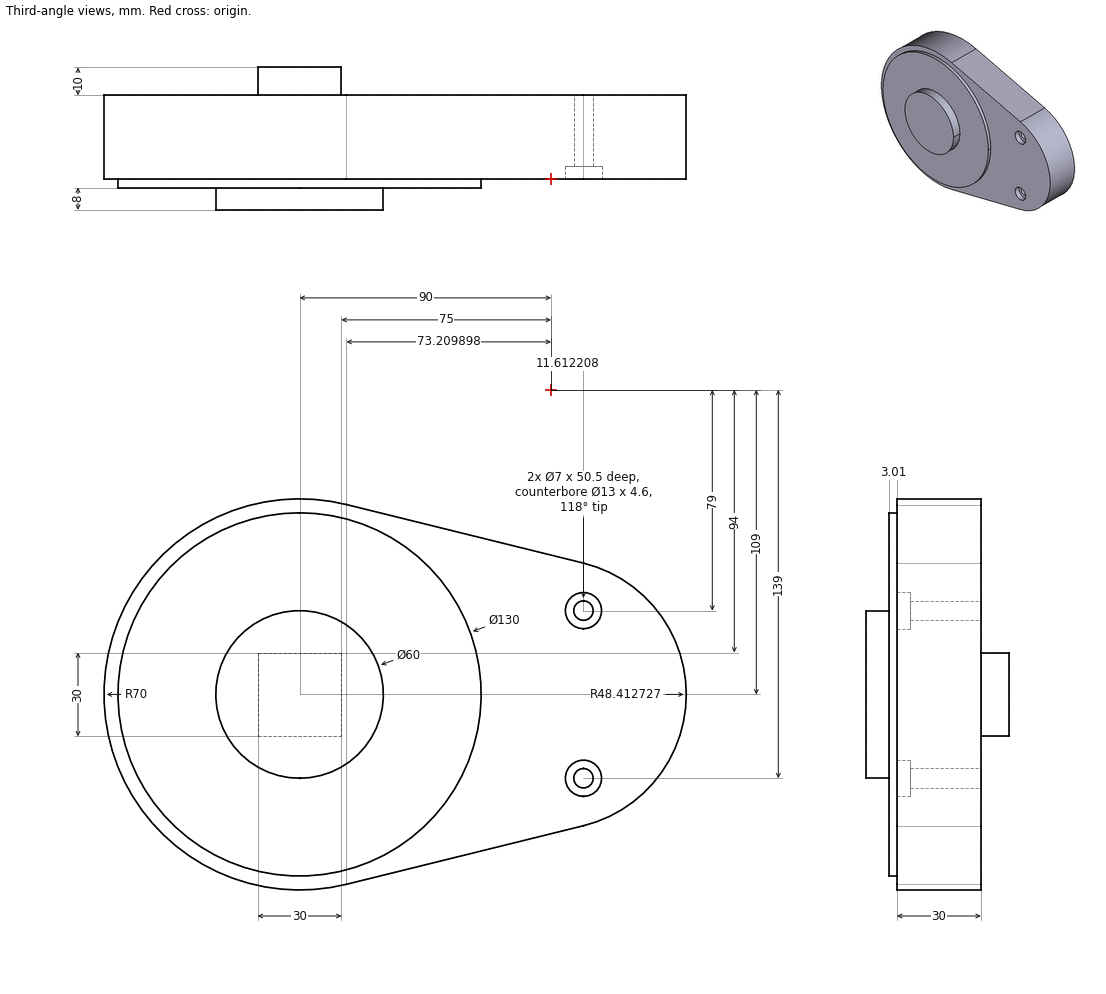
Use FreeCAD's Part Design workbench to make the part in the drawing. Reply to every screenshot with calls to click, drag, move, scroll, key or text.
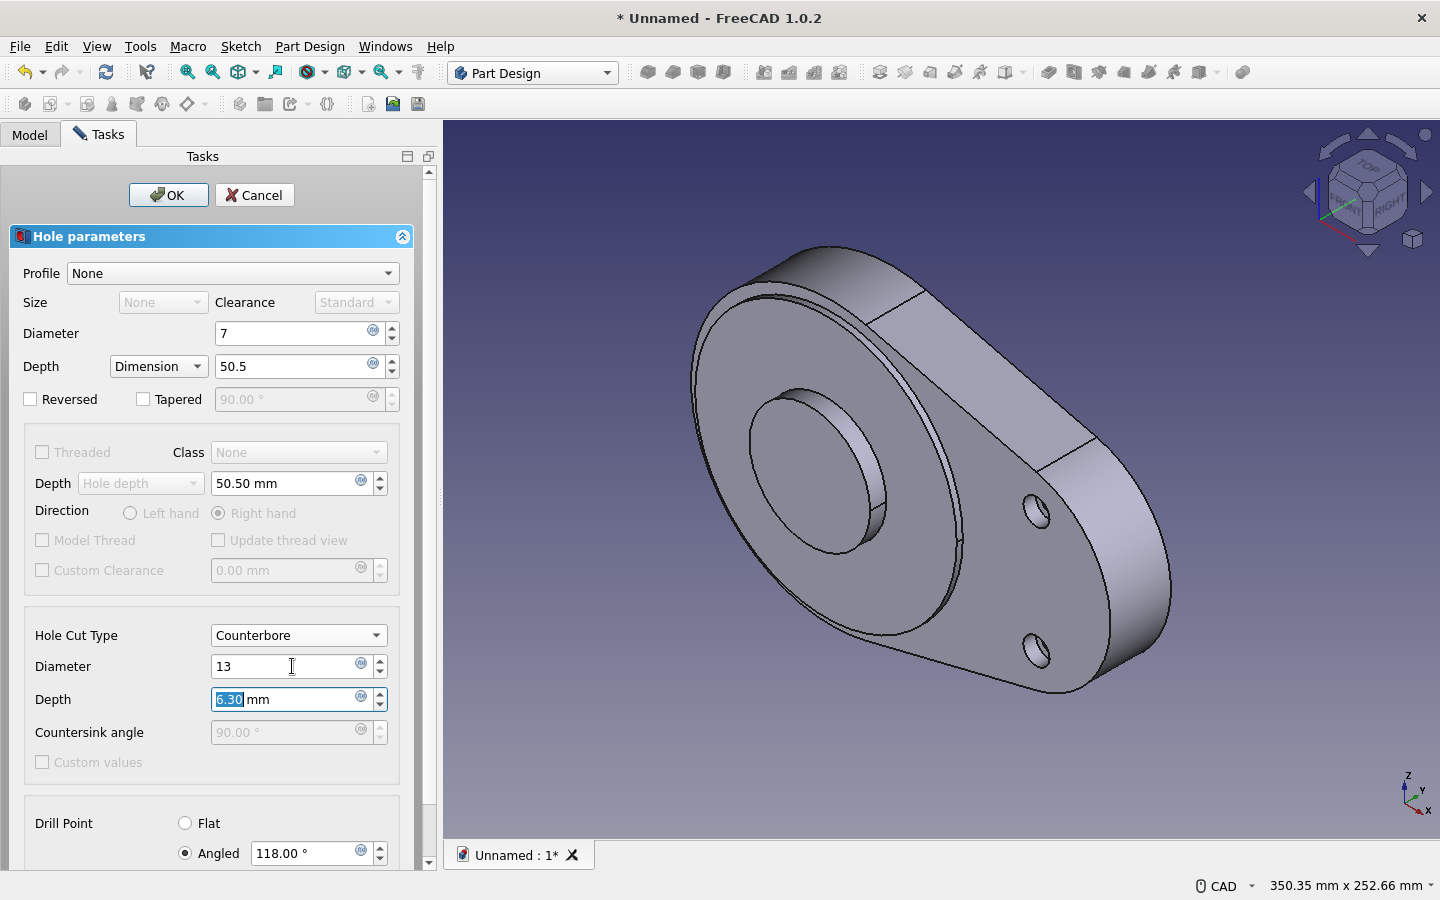
text(4.6)
key(Tab)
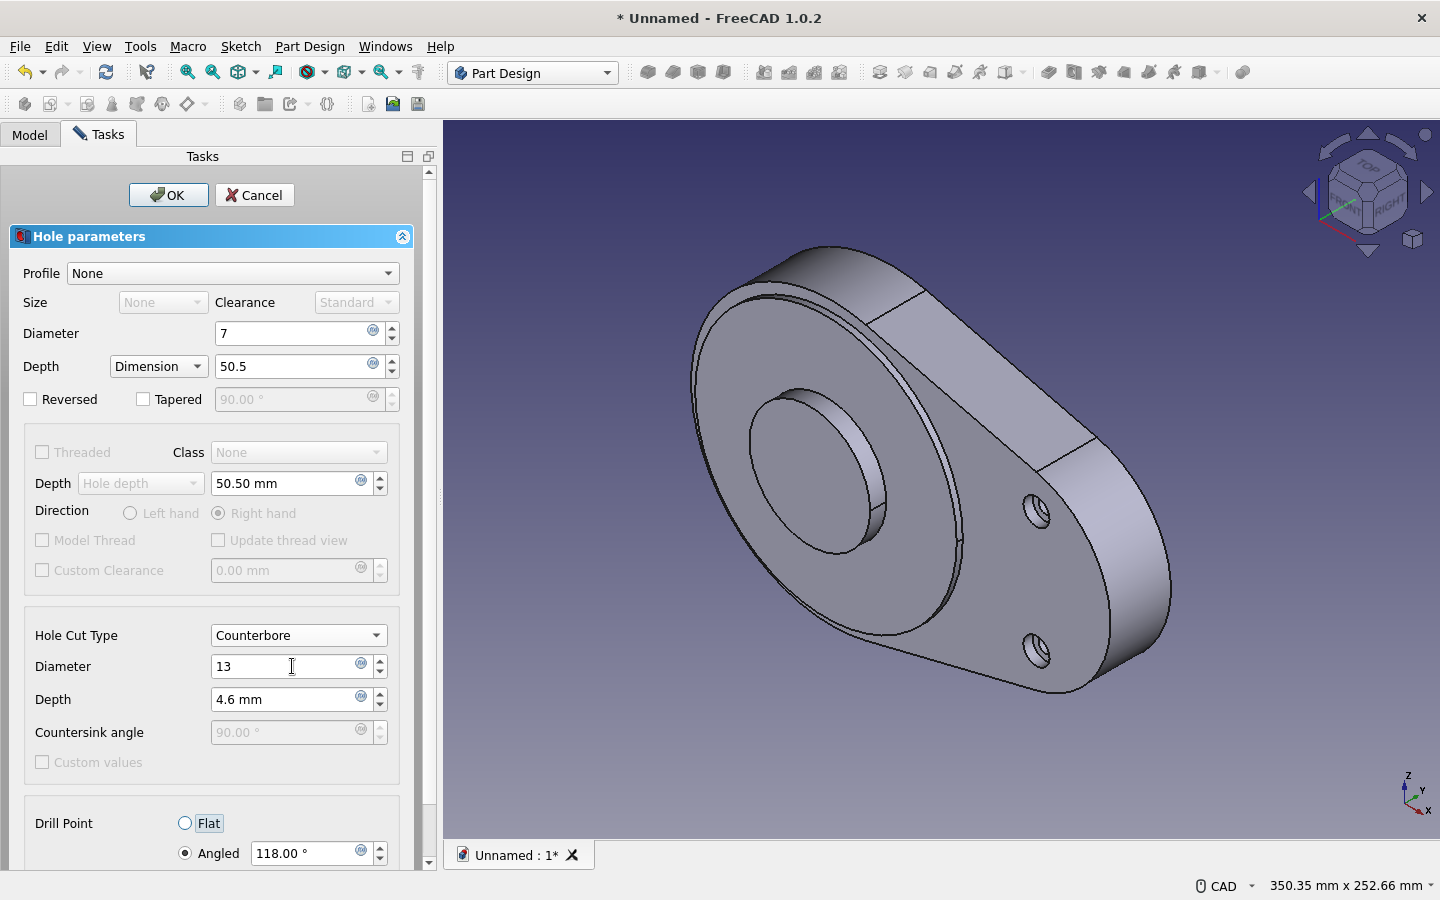
click(169, 195)